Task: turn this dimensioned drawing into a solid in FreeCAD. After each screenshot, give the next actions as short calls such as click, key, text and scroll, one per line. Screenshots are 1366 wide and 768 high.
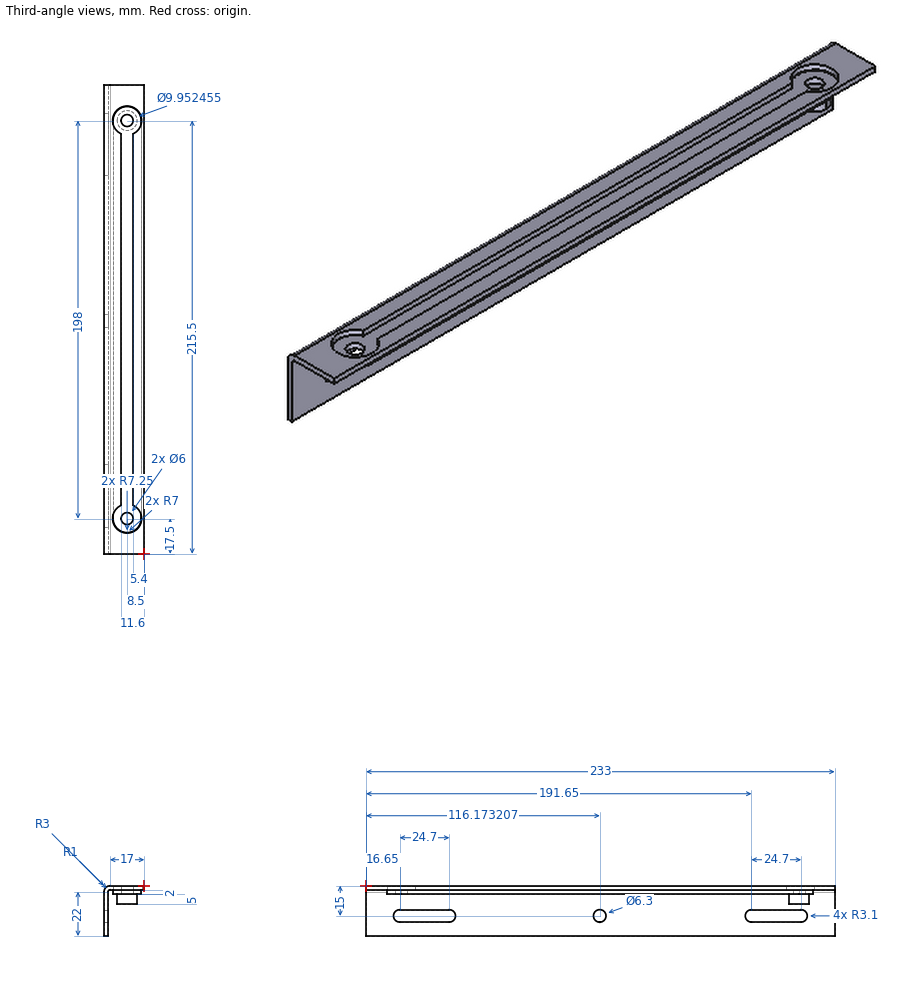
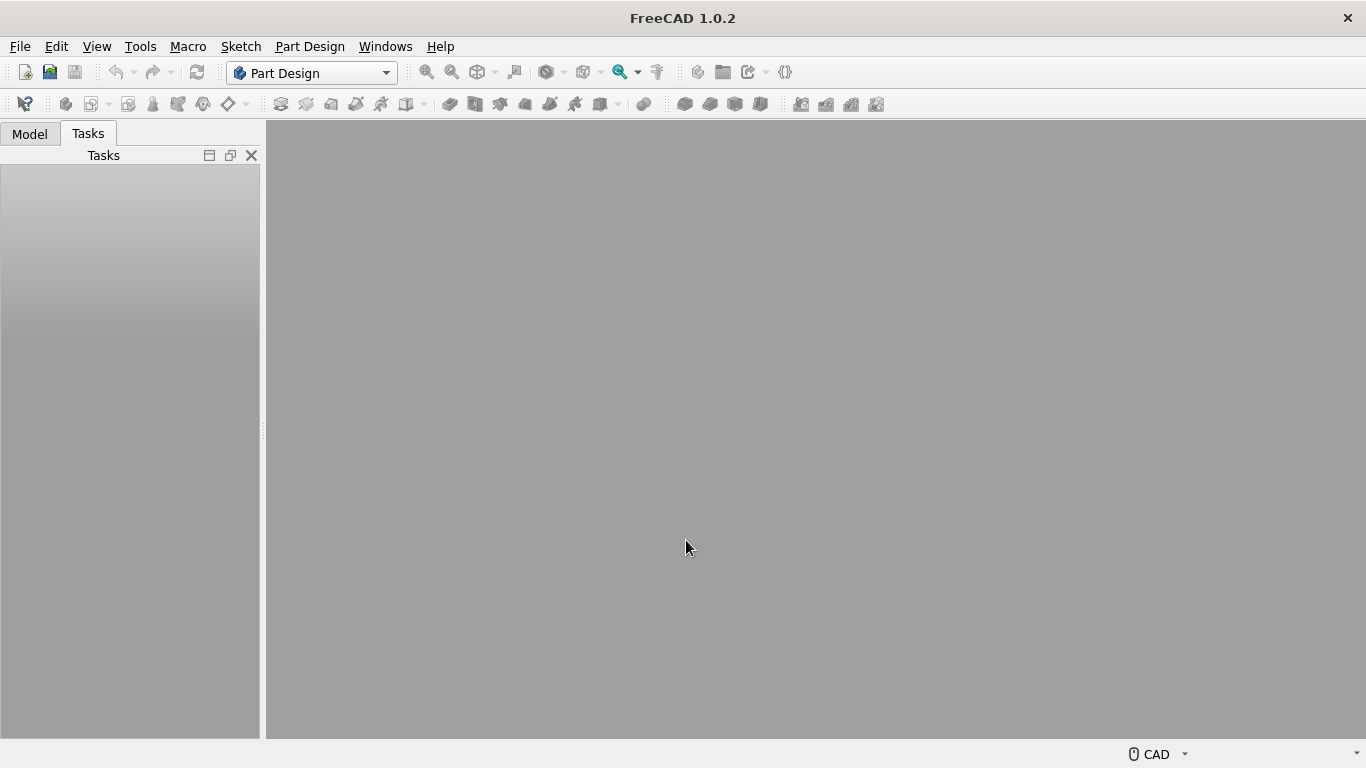
click(25, 72)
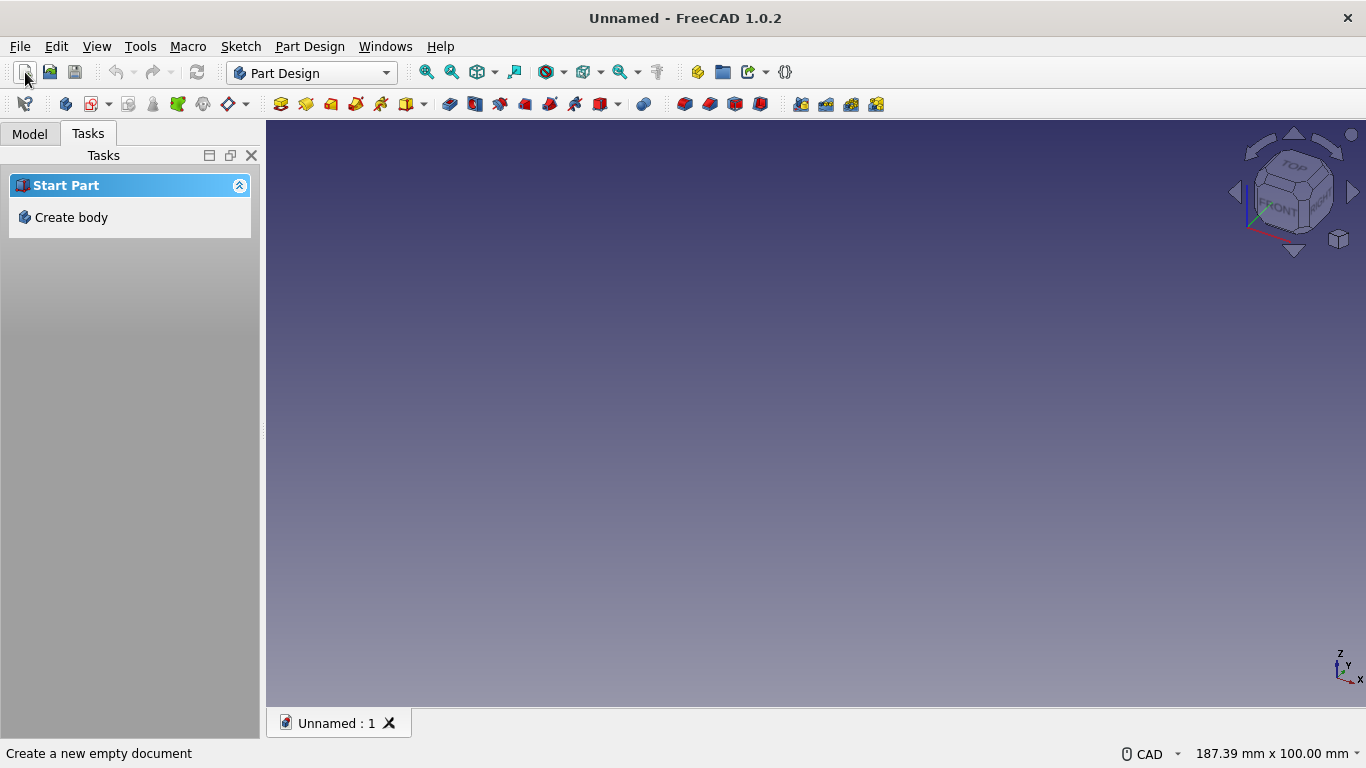
click(90, 104)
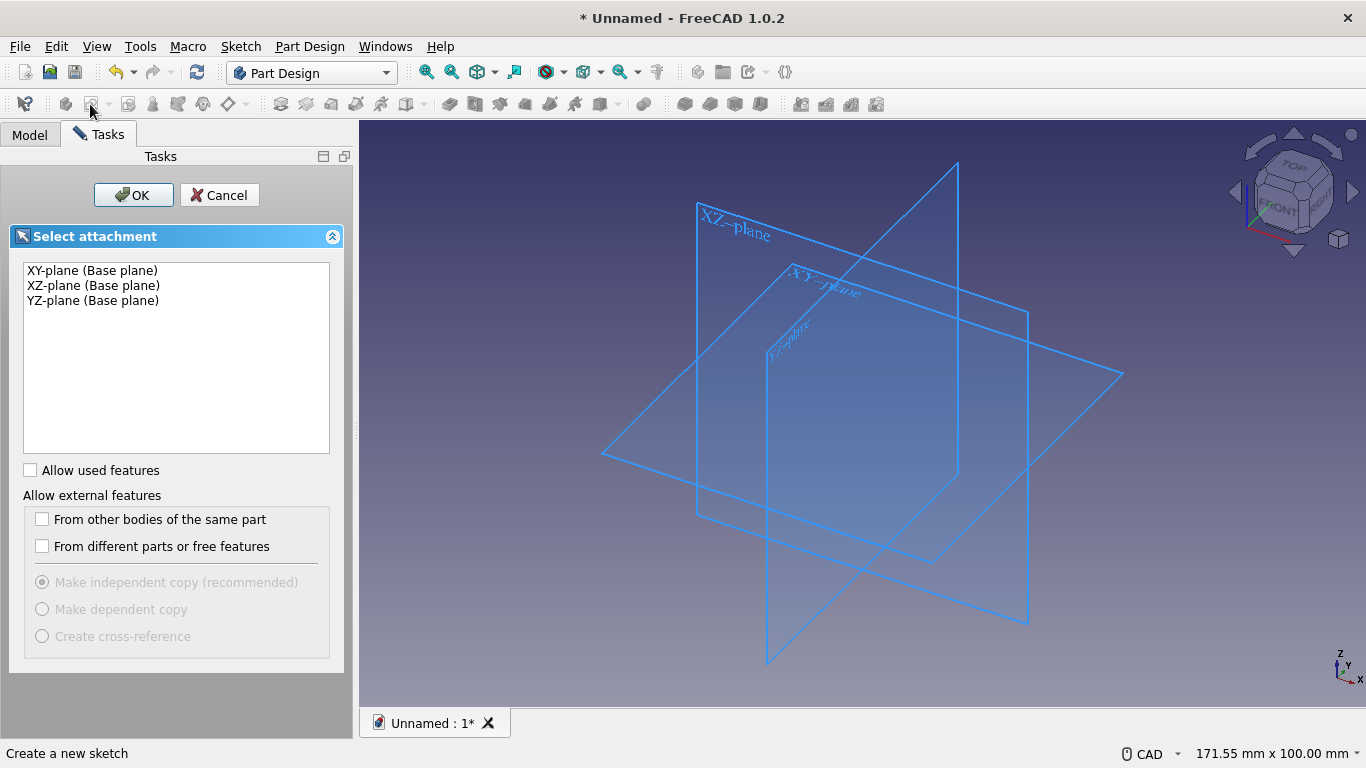
click(84, 286)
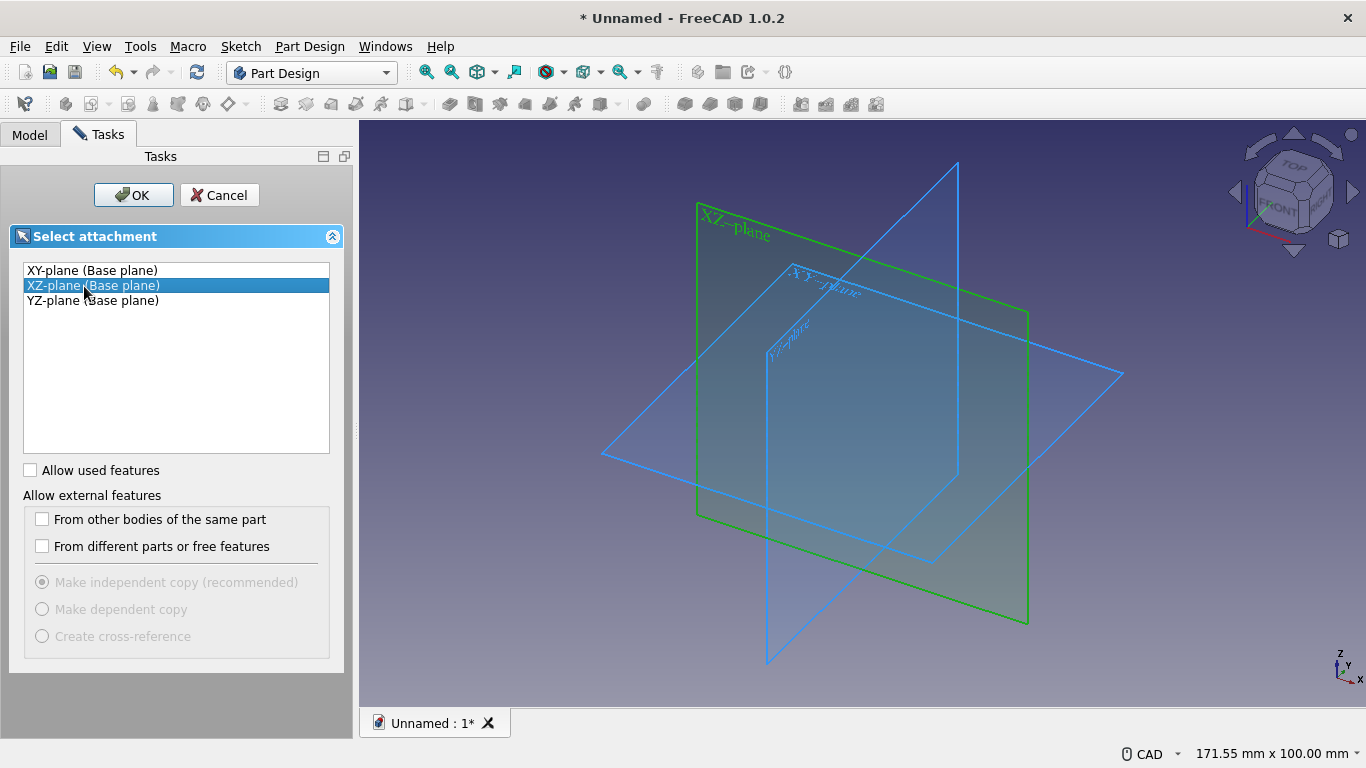
click(134, 195)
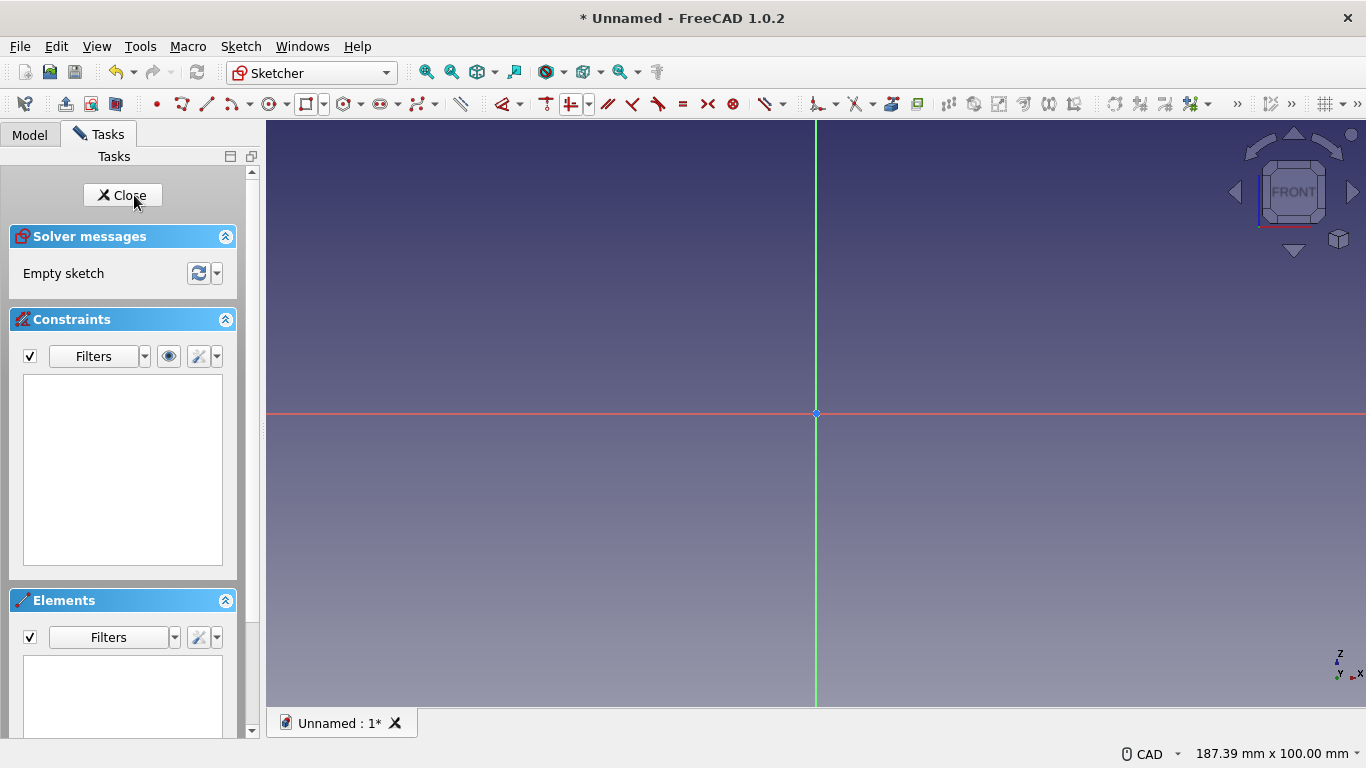
scroll(763, 530, up, 5)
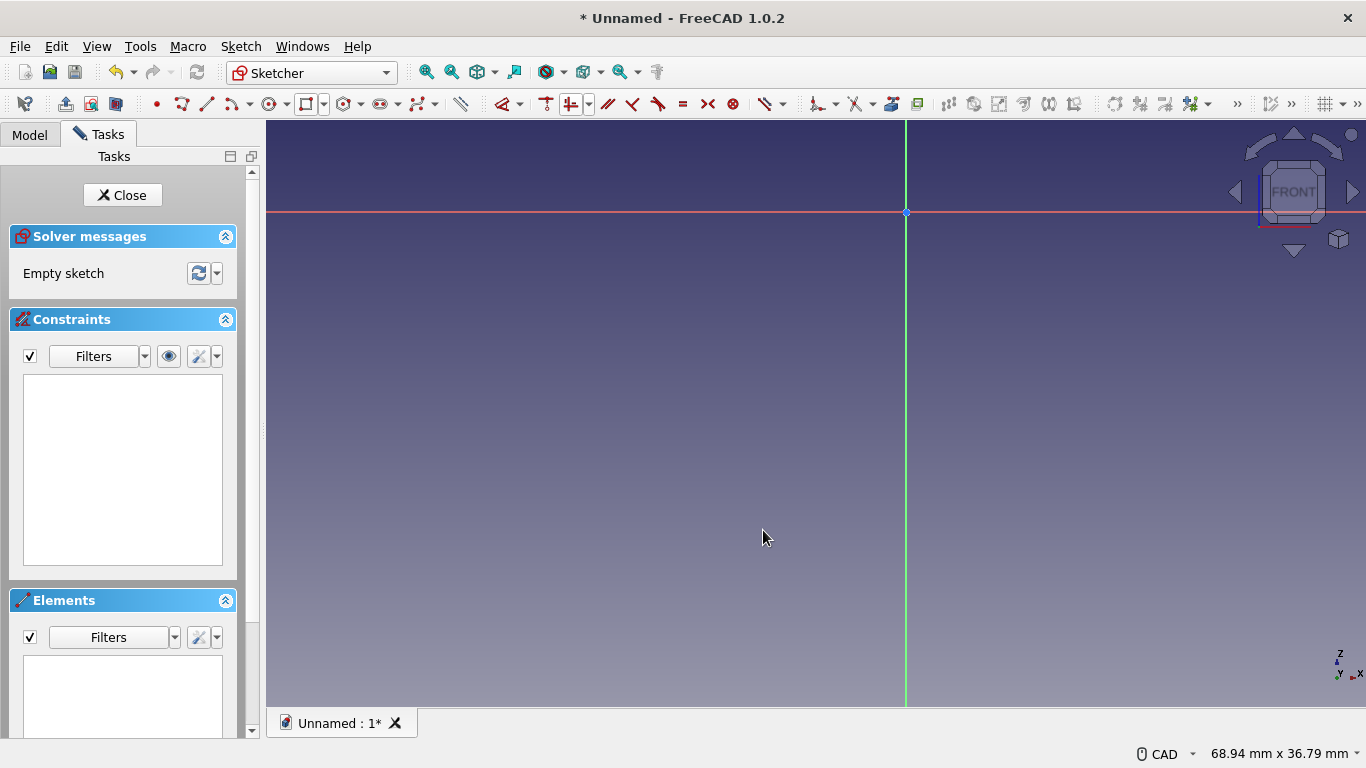
click(182, 104)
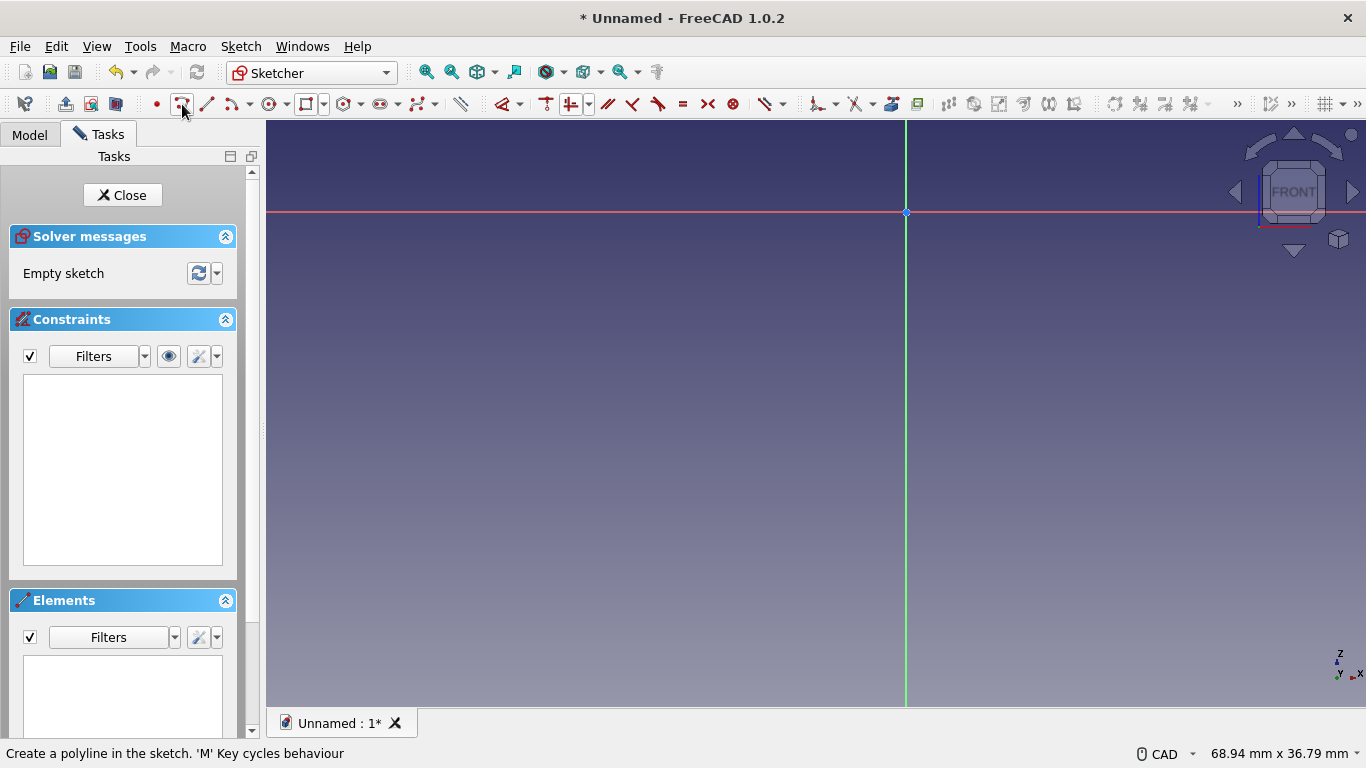
click(635, 212)
click(906, 212)
click(897, 244)
click(635, 244)
right_click(635, 244)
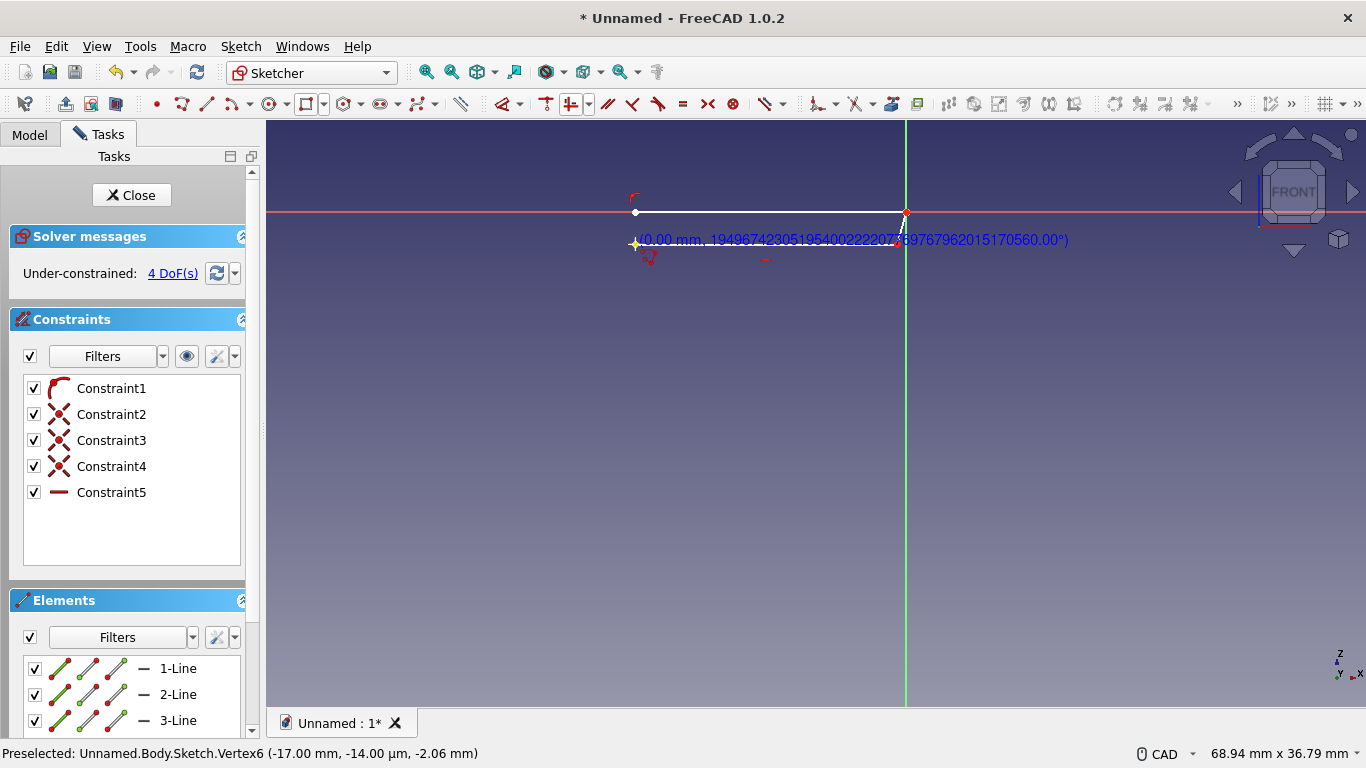
click(619, 260)
click(619, 611)
click(587, 611)
click(587, 260)
right_click(587, 260)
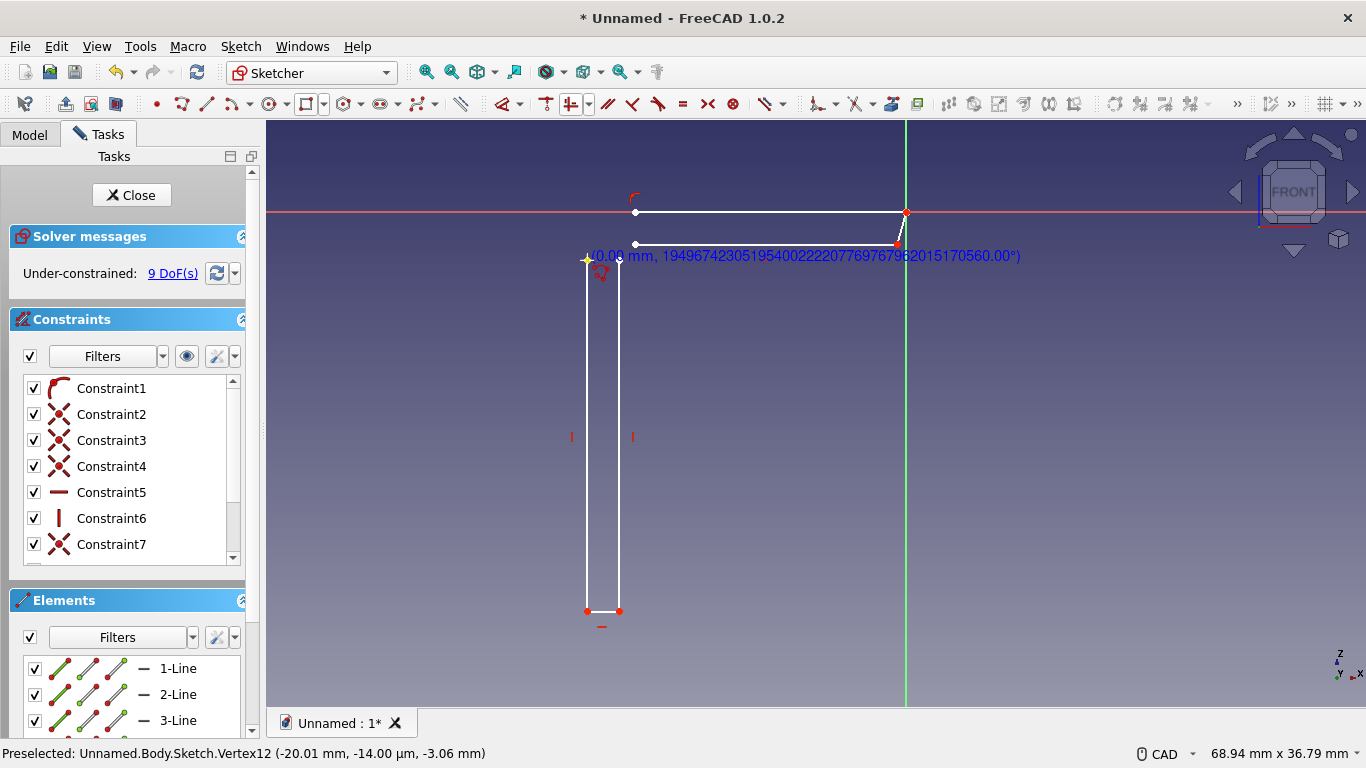
click(250, 104)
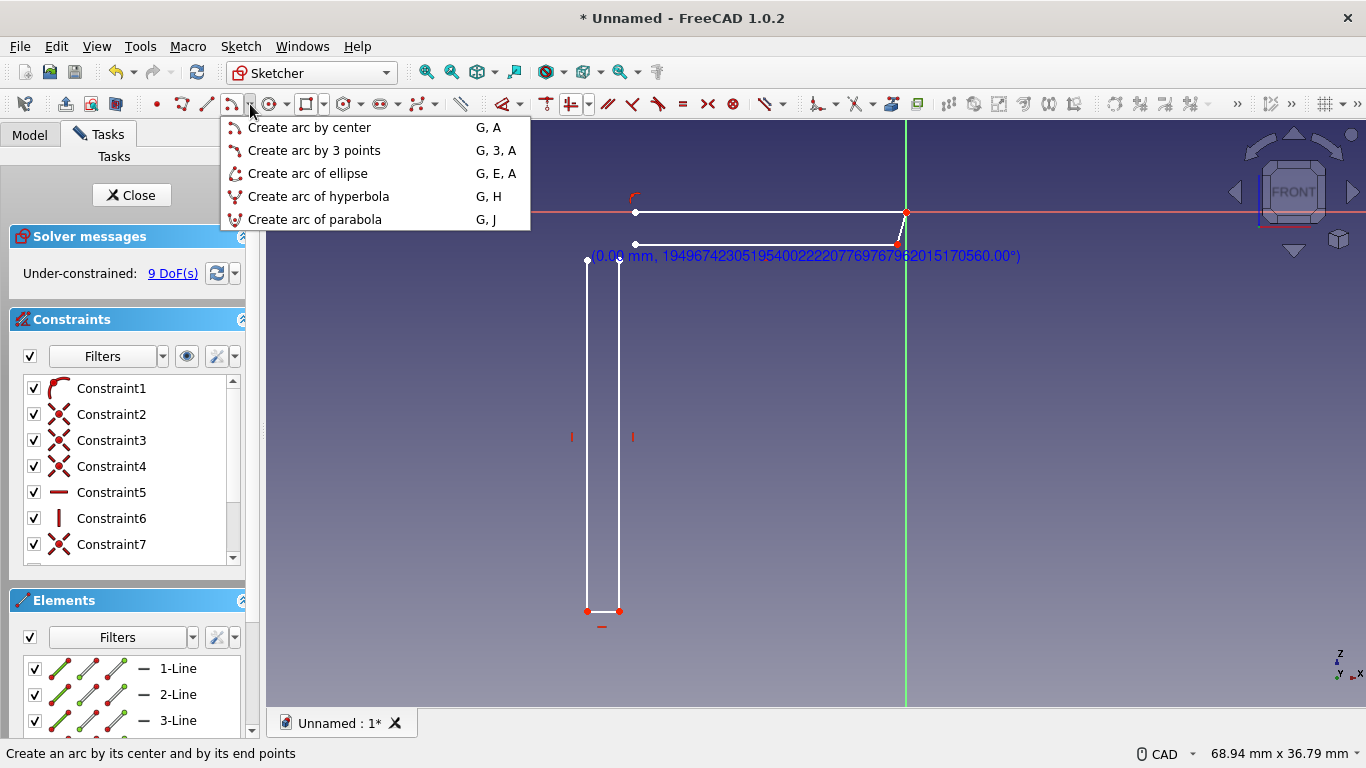
click(376, 150)